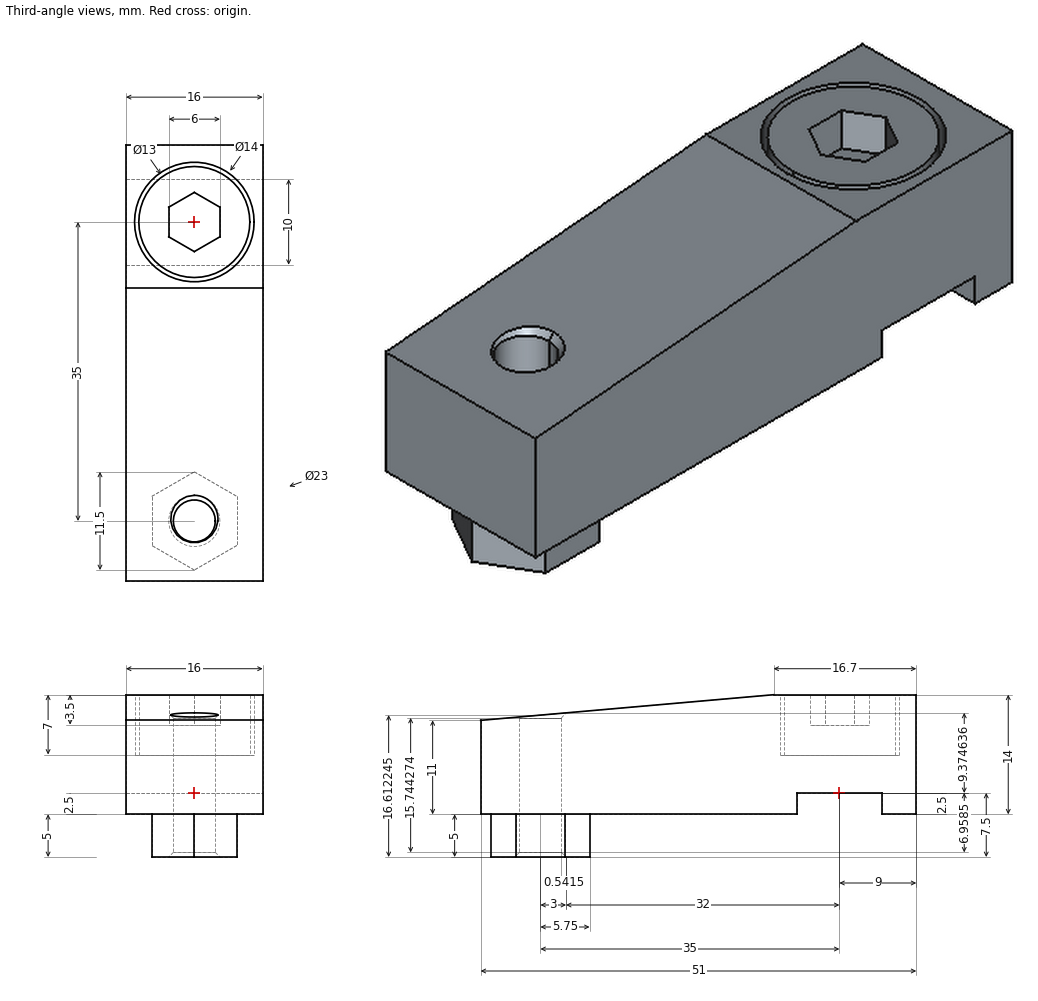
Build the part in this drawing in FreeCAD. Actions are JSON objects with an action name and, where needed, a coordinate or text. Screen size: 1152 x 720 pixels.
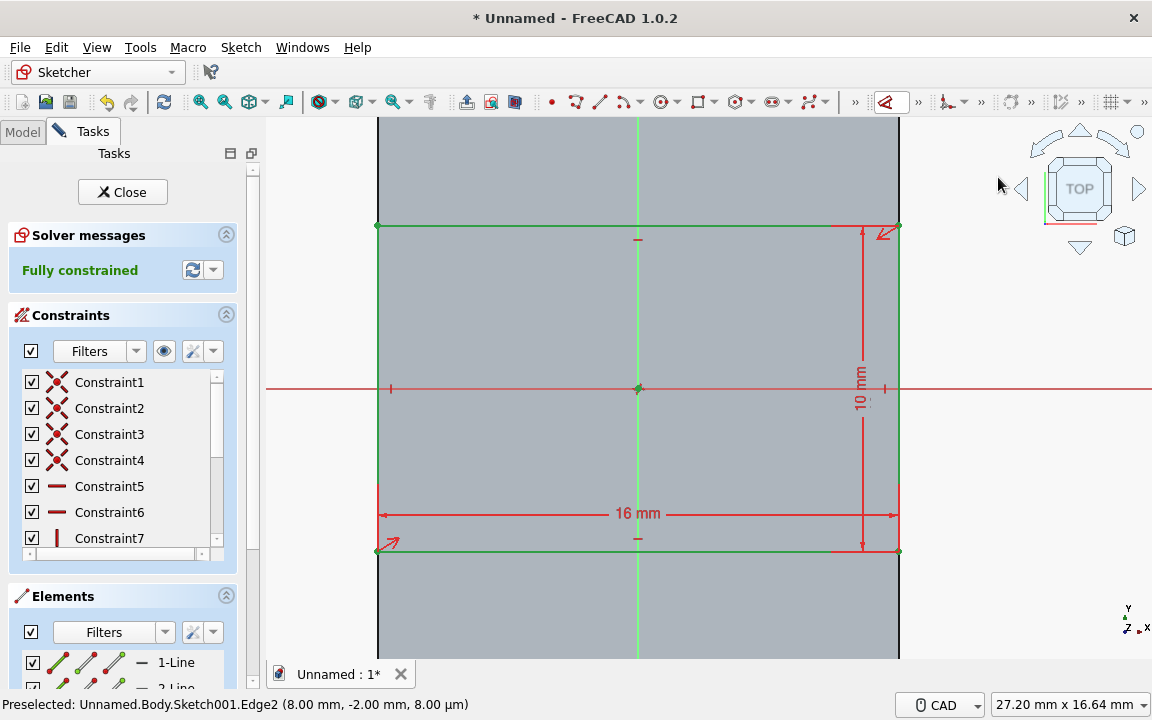
{"action": "left_click", "coordinate": [123, 192]}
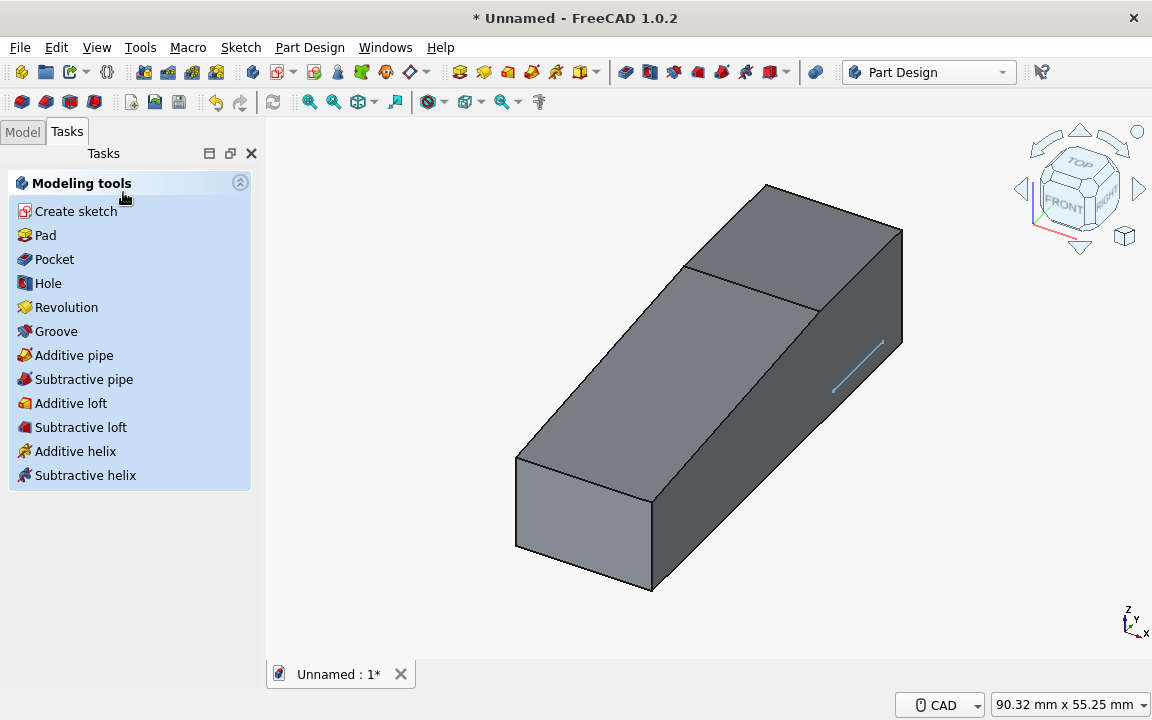
{"action": "left_click", "coordinate": [626, 72]}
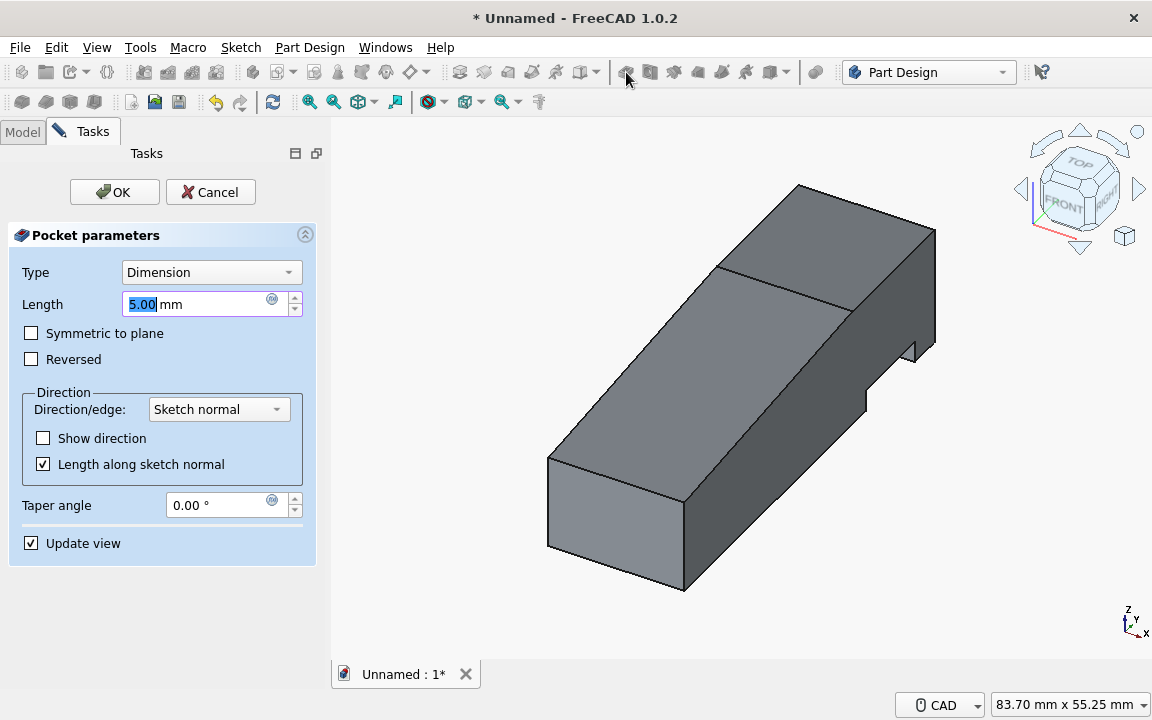
{"action": "type", "text": "2.5"}
{"action": "key", "text": "Tab"}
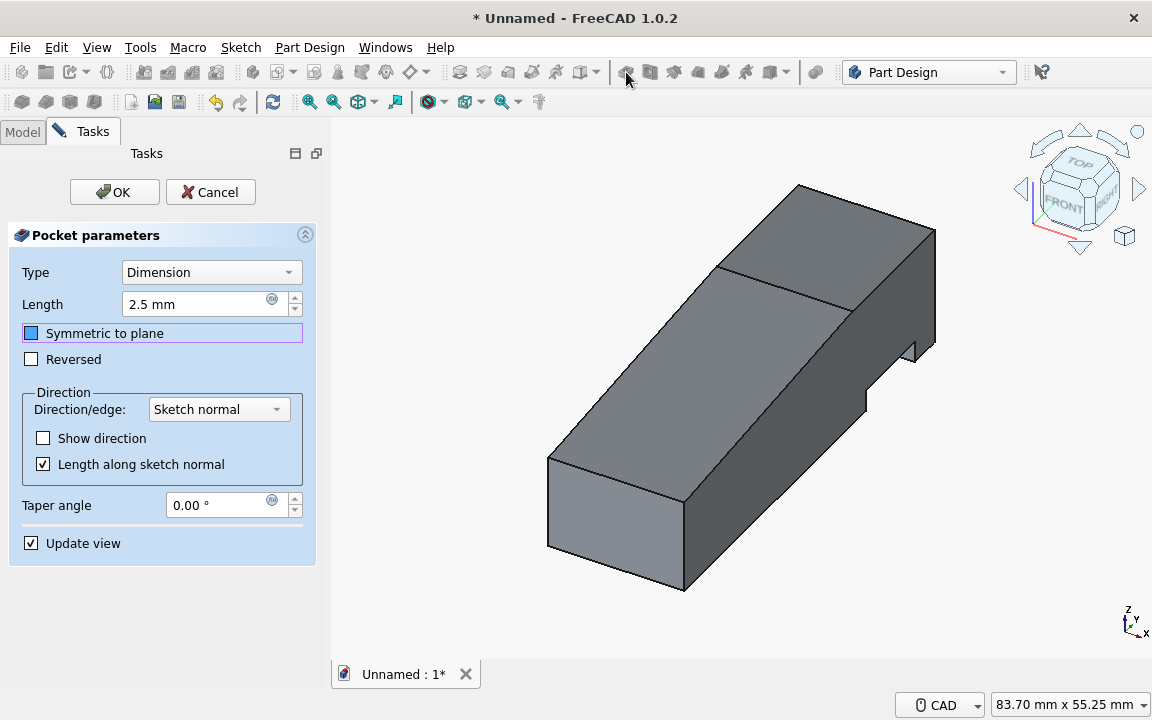
{"action": "left_click", "coordinate": [115, 192]}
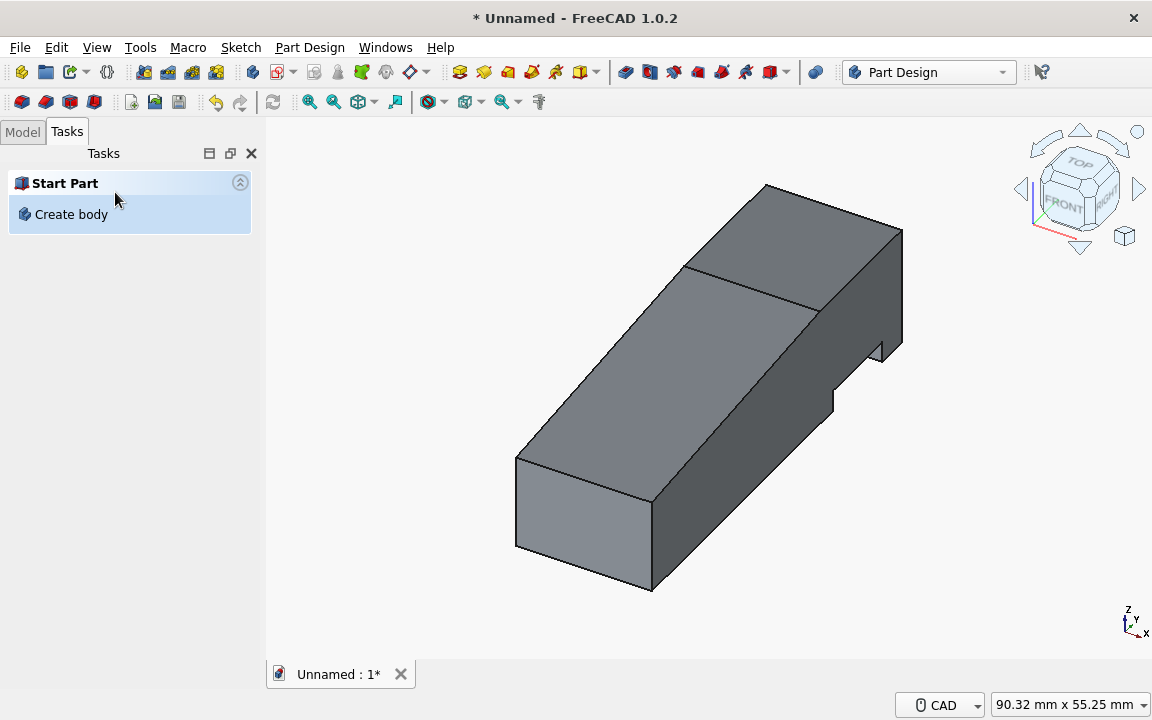
{"action": "left_click", "coordinate": [278, 72]}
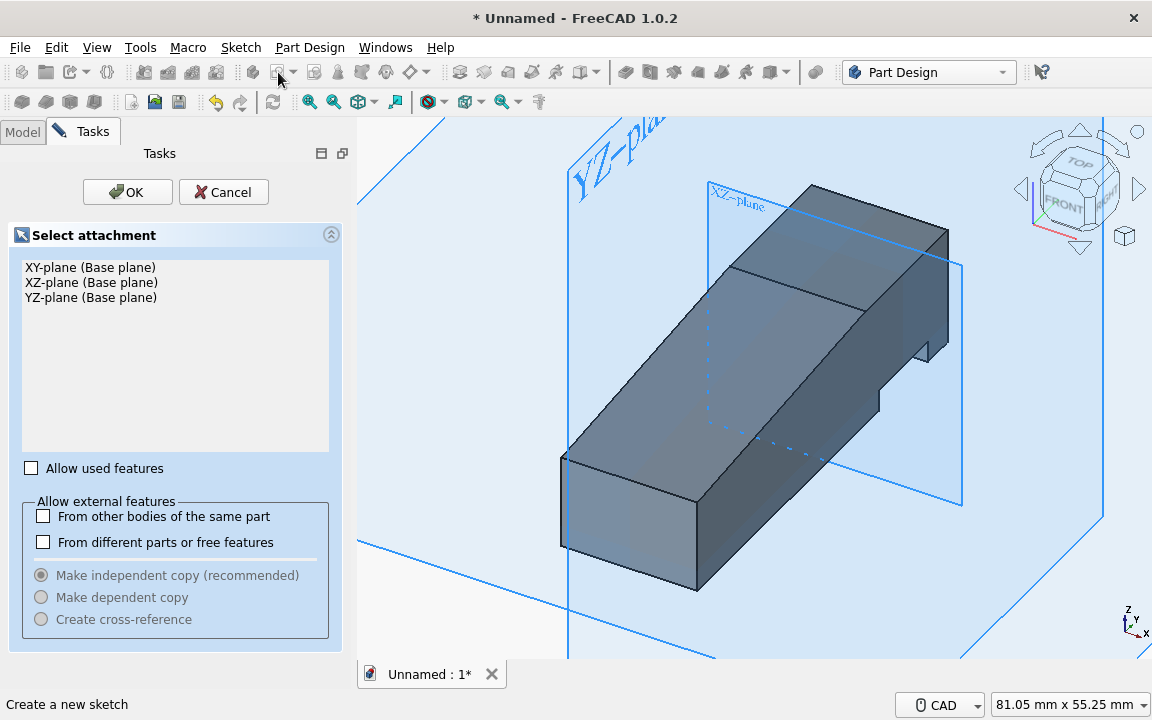
{"action": "left_click", "coordinate": [82, 298]}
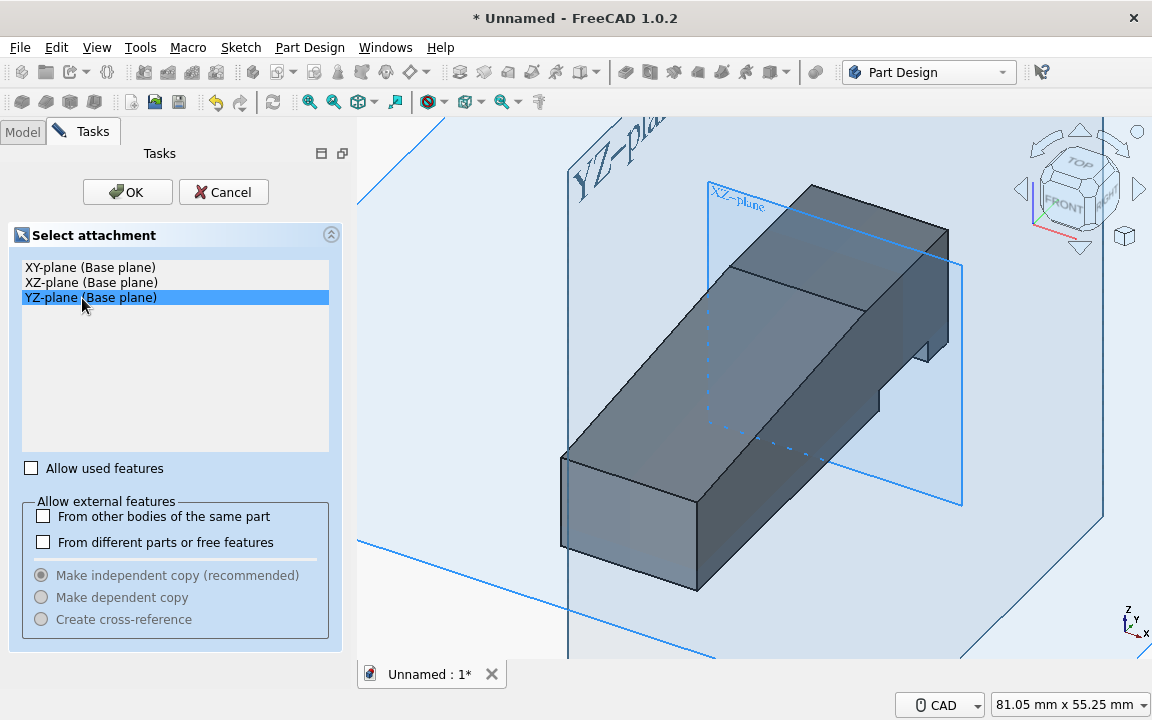
{"action": "left_click", "coordinate": [128, 192]}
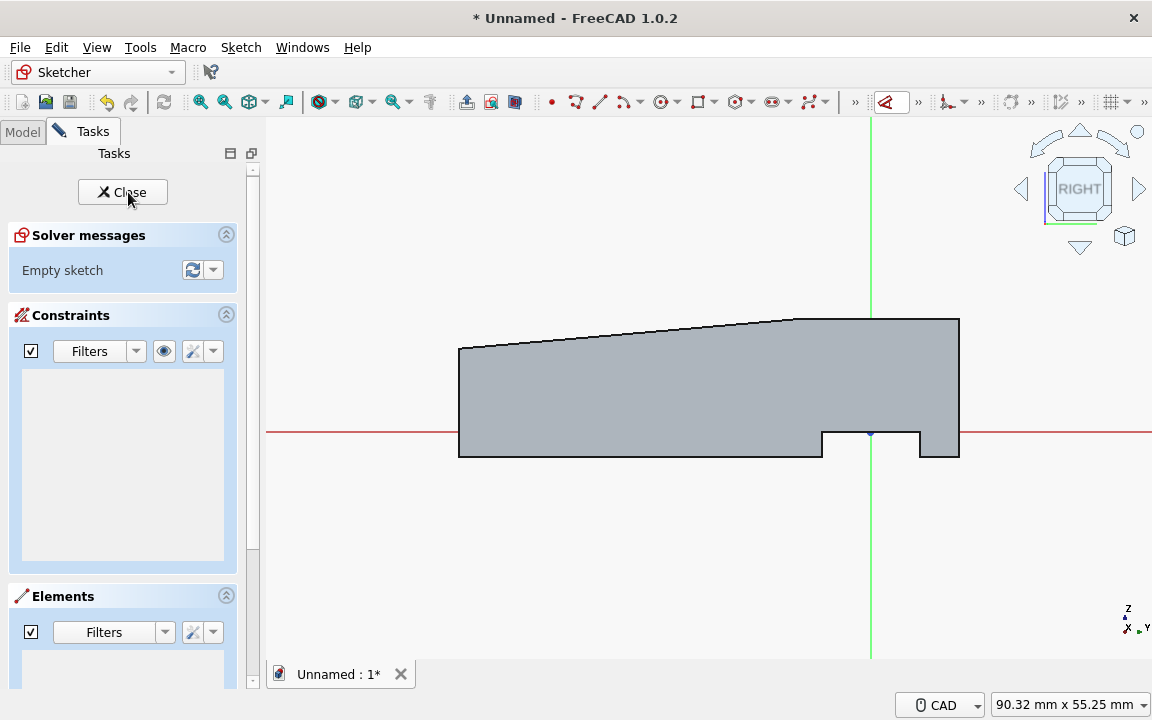
{"action": "left_click", "coordinate": [516, 102]}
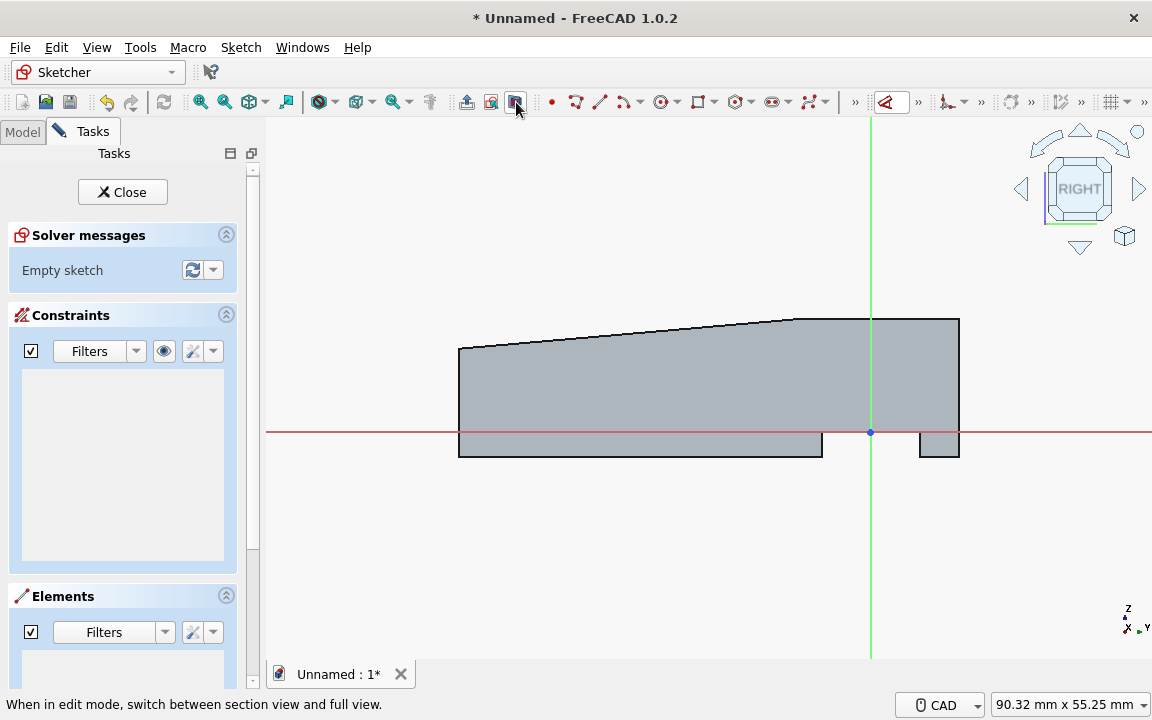
{"action": "scroll", "coordinate": [534, 492], "scroll_direction": "up", "scroll_amount": 8}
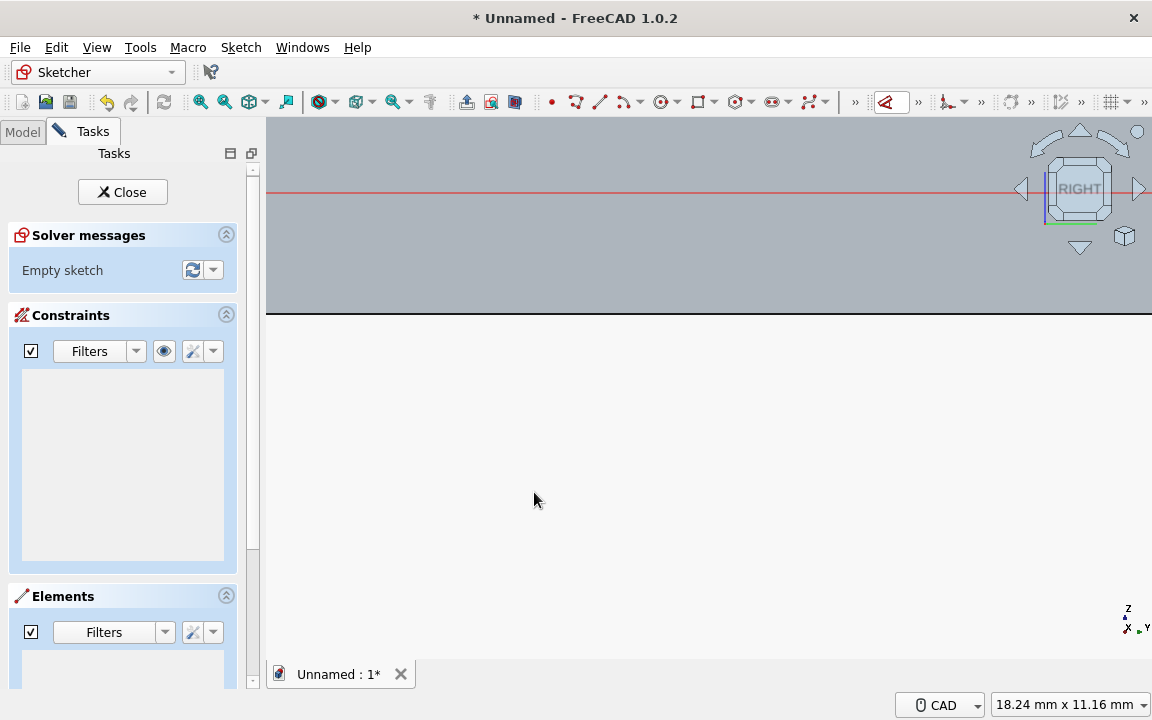
{"action": "left_click", "coordinate": [698, 102]}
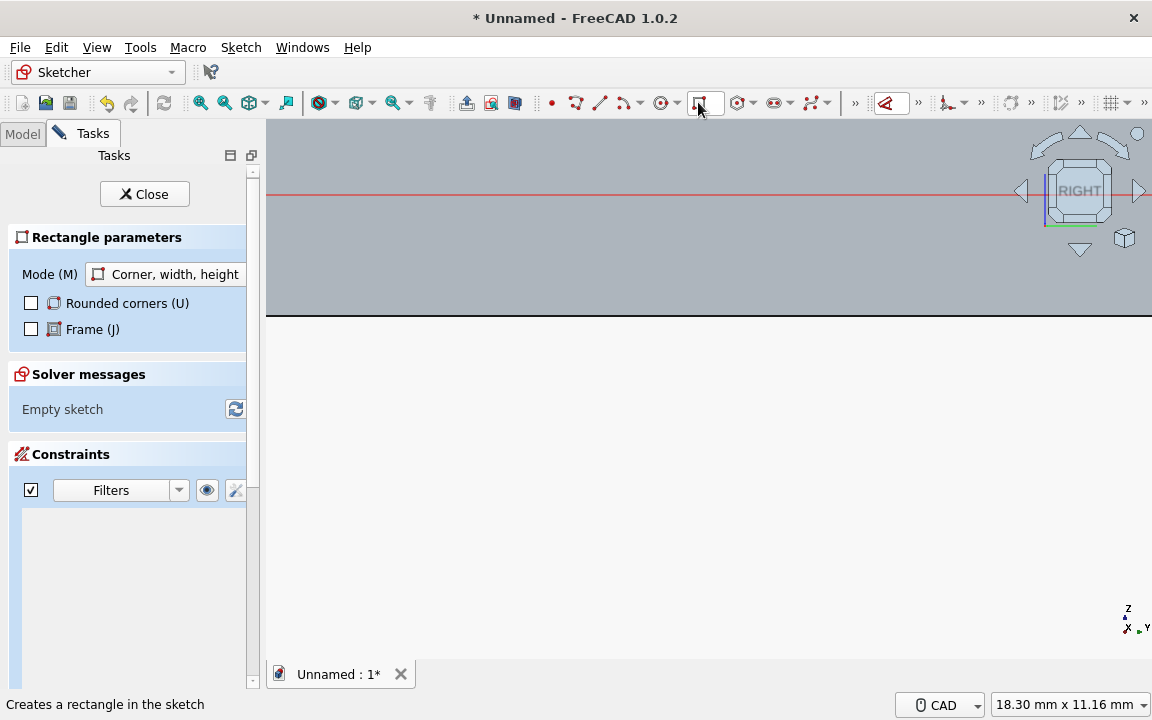
{"action": "left_click", "coordinate": [502, 316]}
{"action": "left_click", "coordinate": [780, 558]}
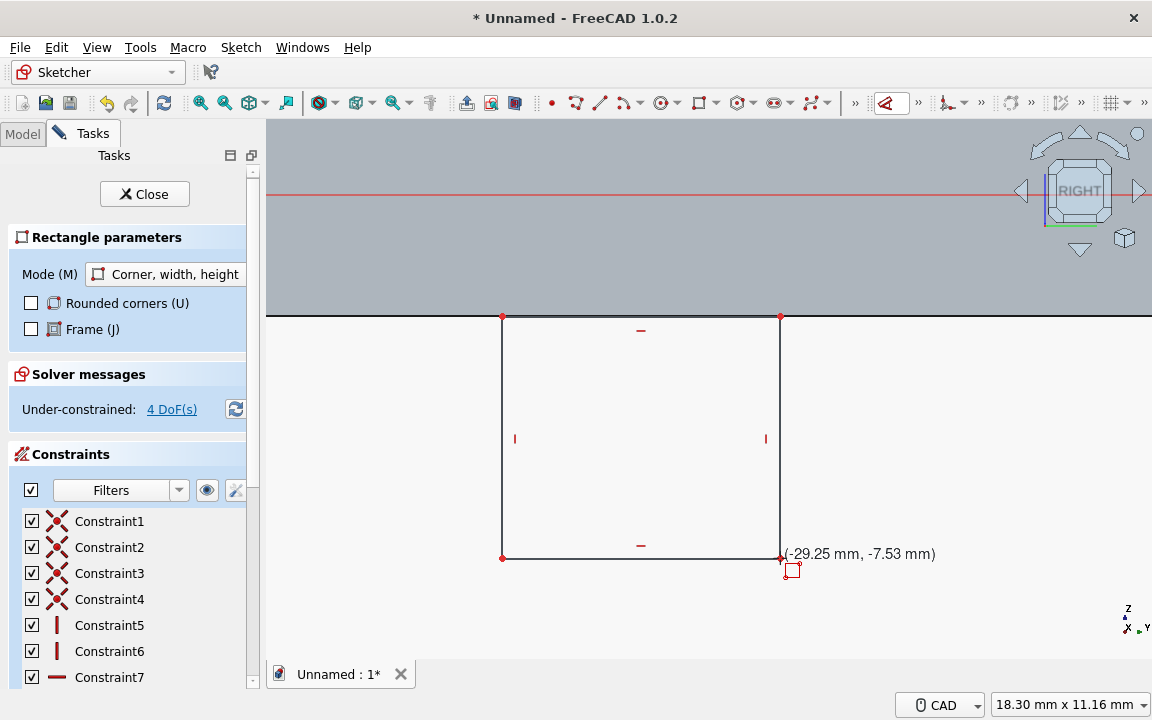
{"action": "left_click", "coordinate": [600, 104]}